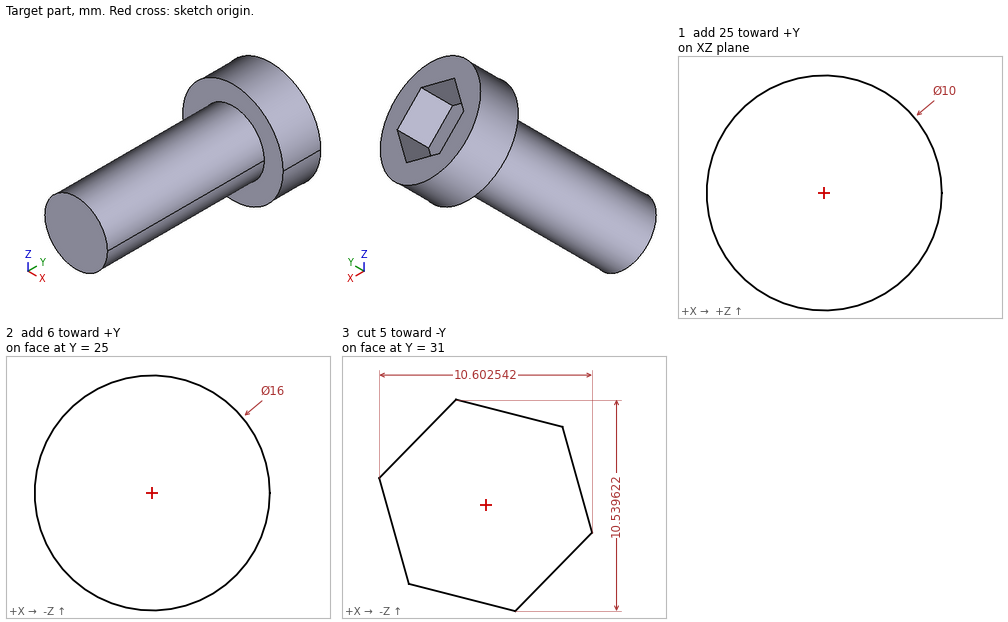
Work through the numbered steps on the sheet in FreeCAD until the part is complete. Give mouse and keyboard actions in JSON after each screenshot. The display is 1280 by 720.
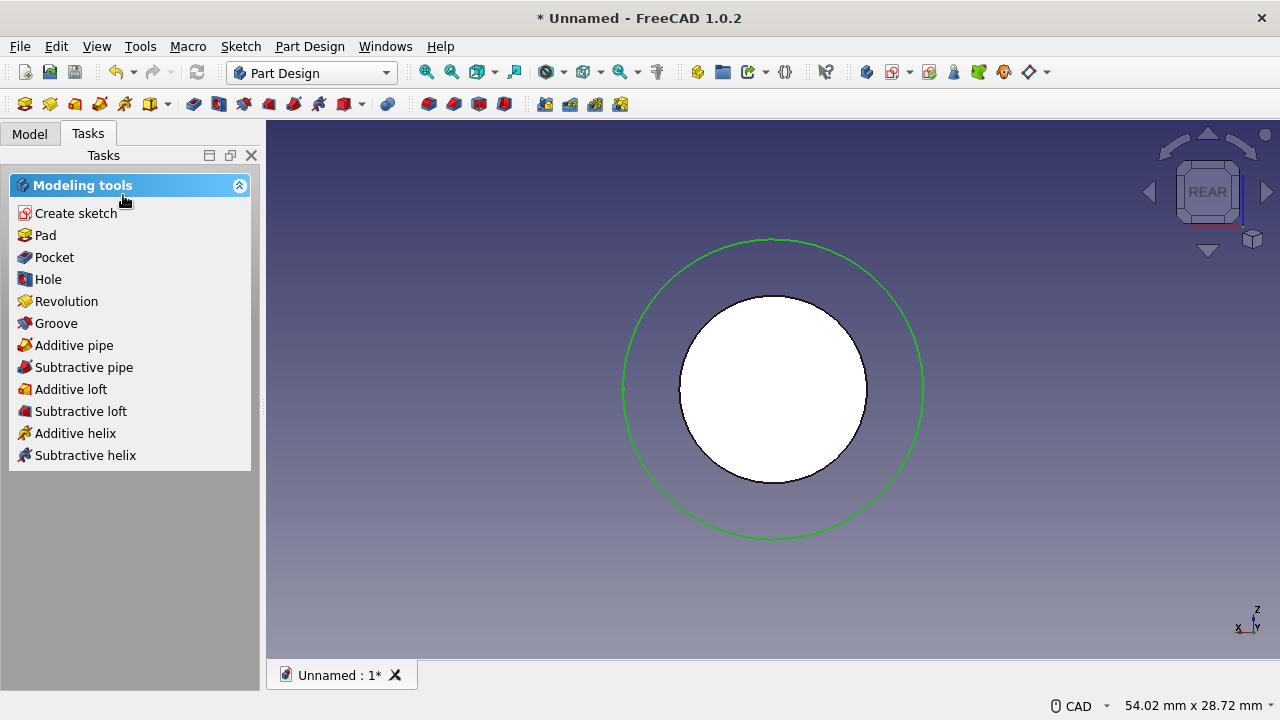
{"action": "left_click", "coordinate": [25, 104]}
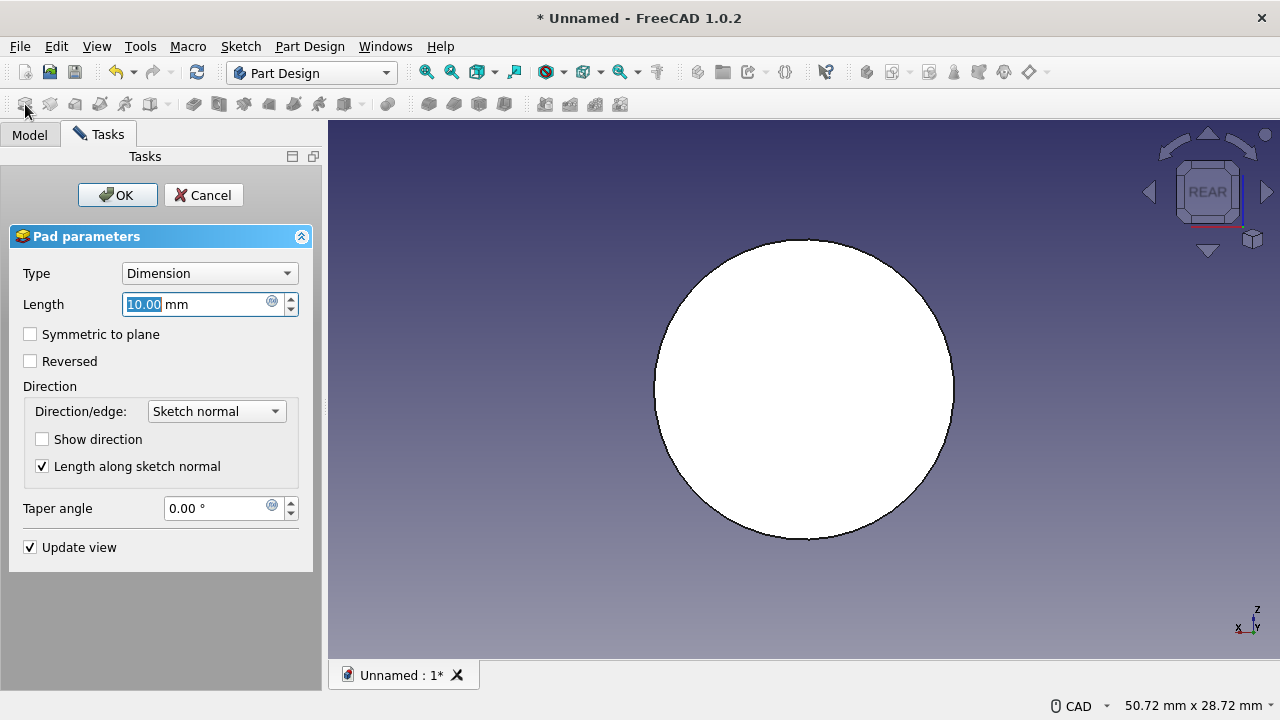
{"action": "type", "text": "6"}
{"action": "key", "text": "Tab"}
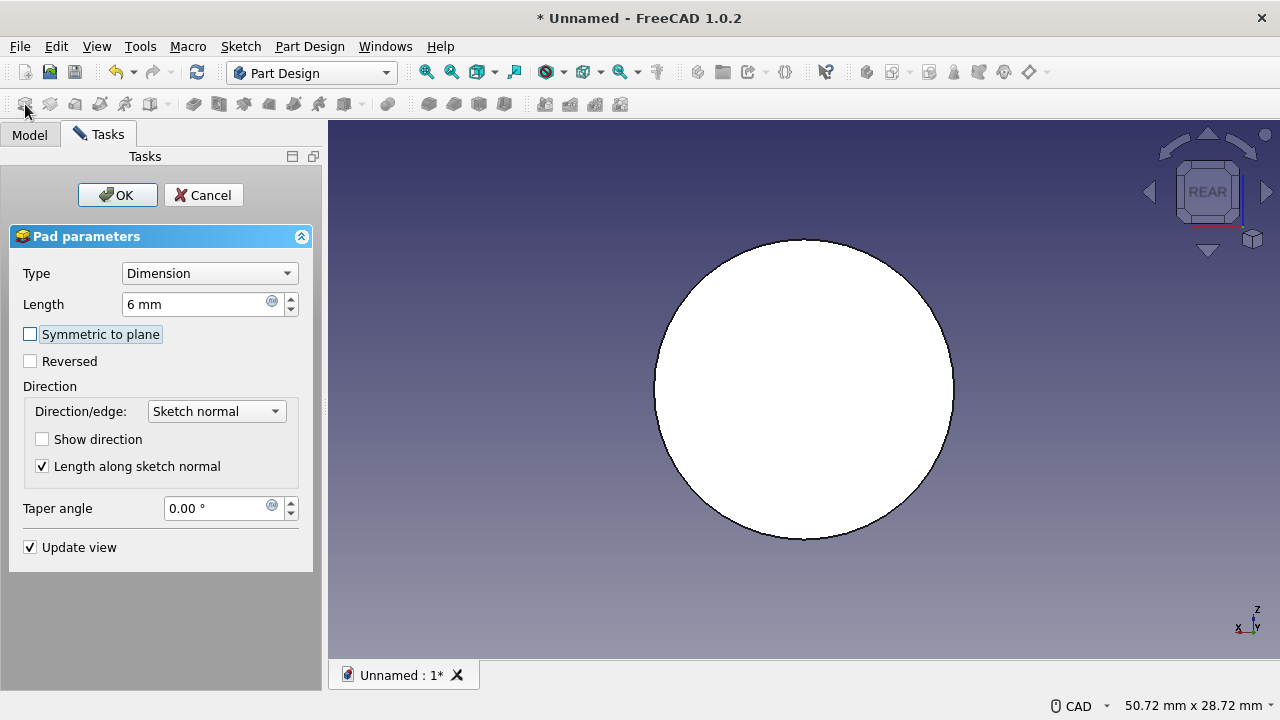
{"action": "left_click", "coordinate": [118, 195]}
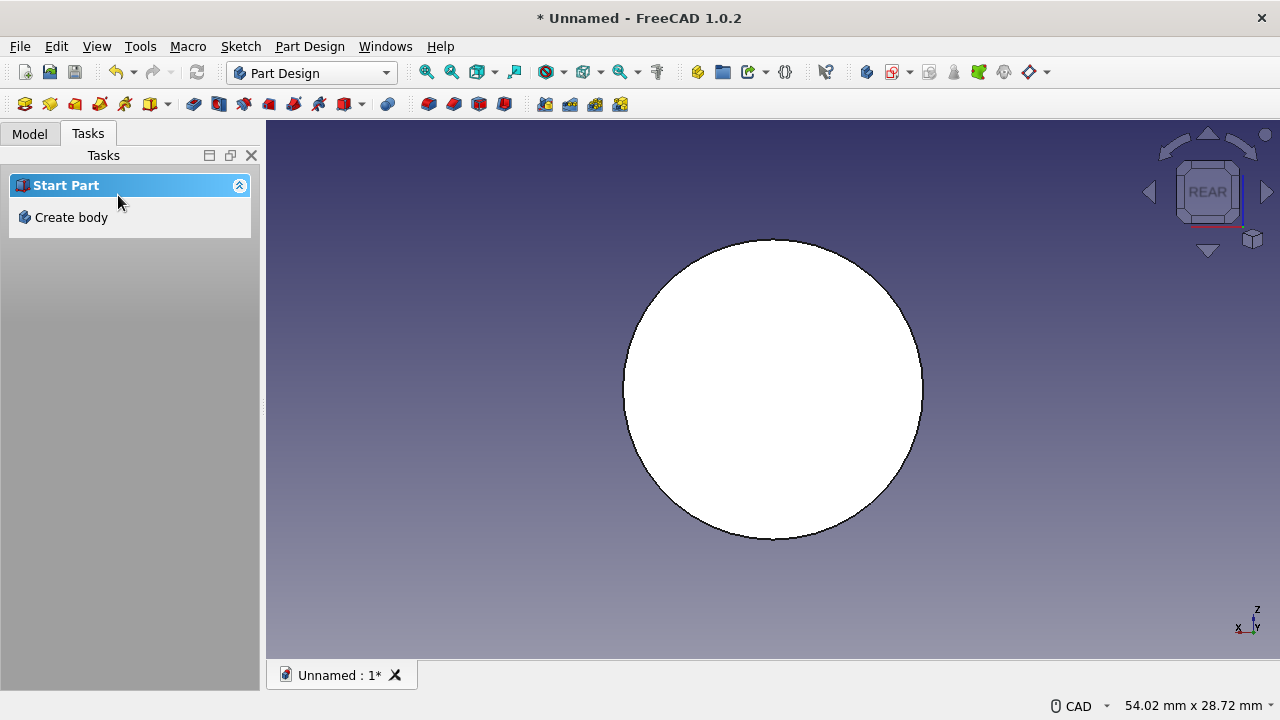
{"action": "left_click", "coordinate": [773, 389]}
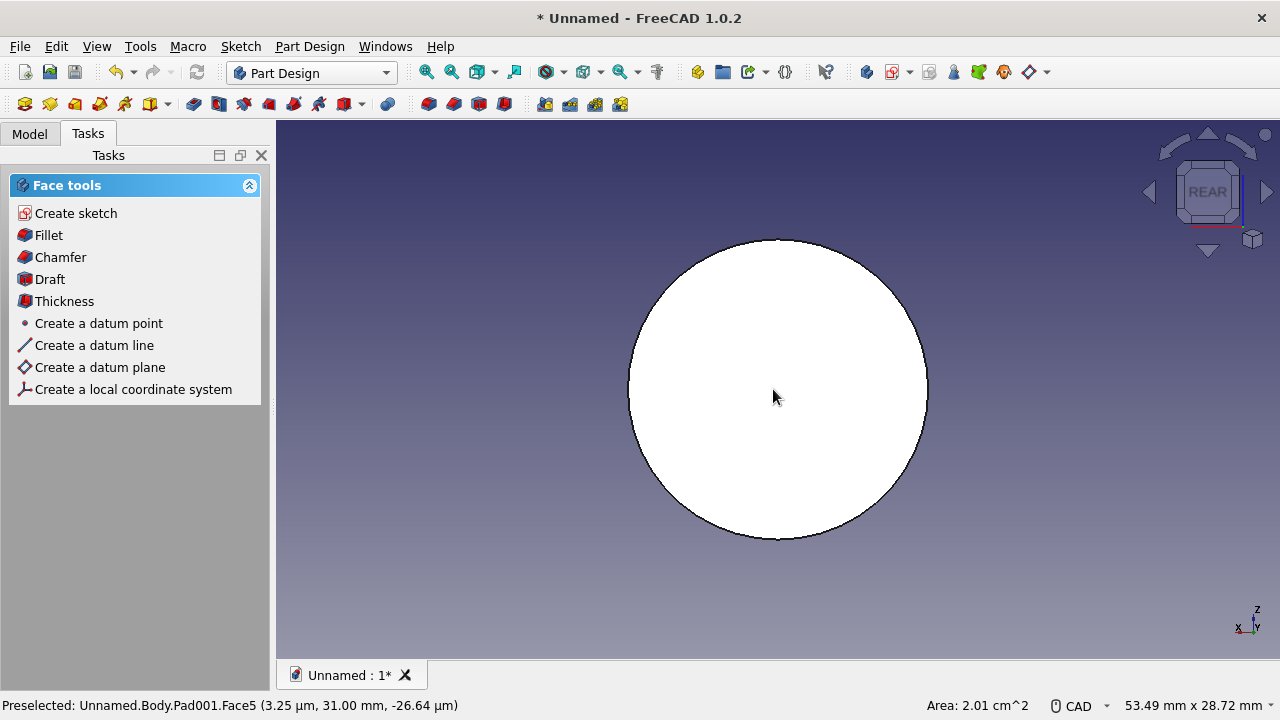
{"action": "left_click", "coordinate": [892, 72]}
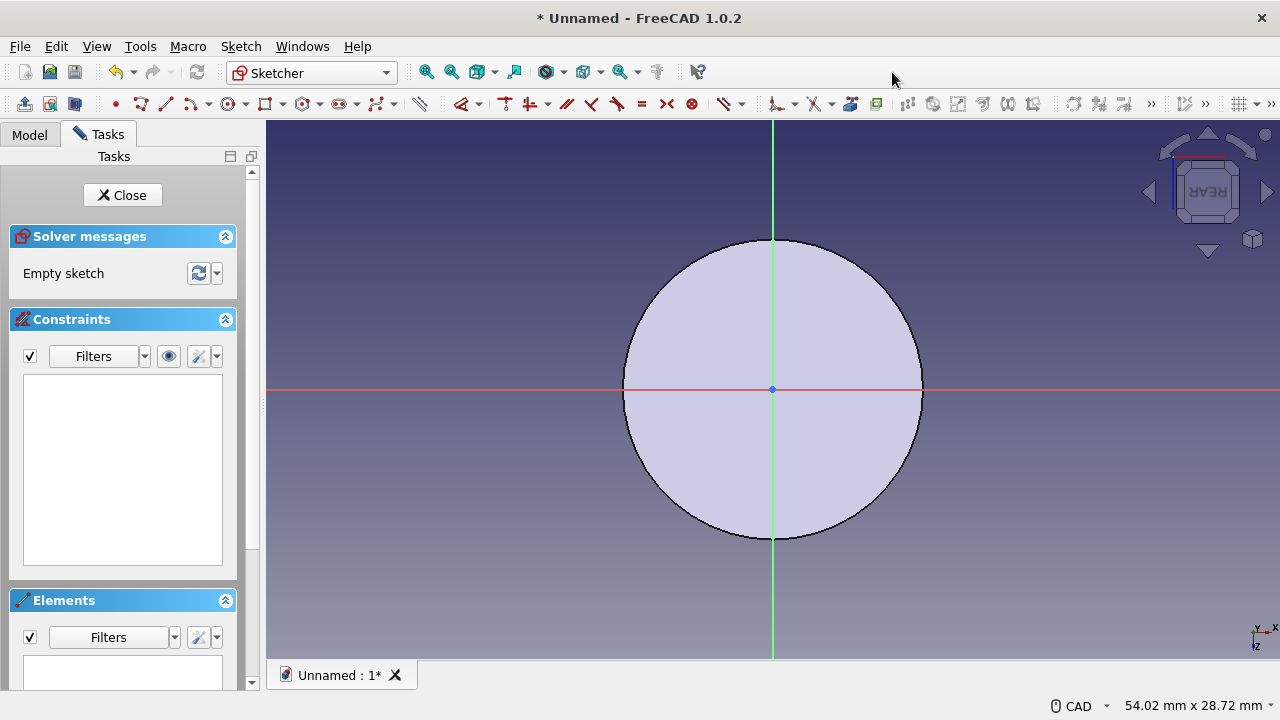
{"action": "scroll", "coordinate": [856, 389], "scroll_direction": "up", "scroll_amount": 3}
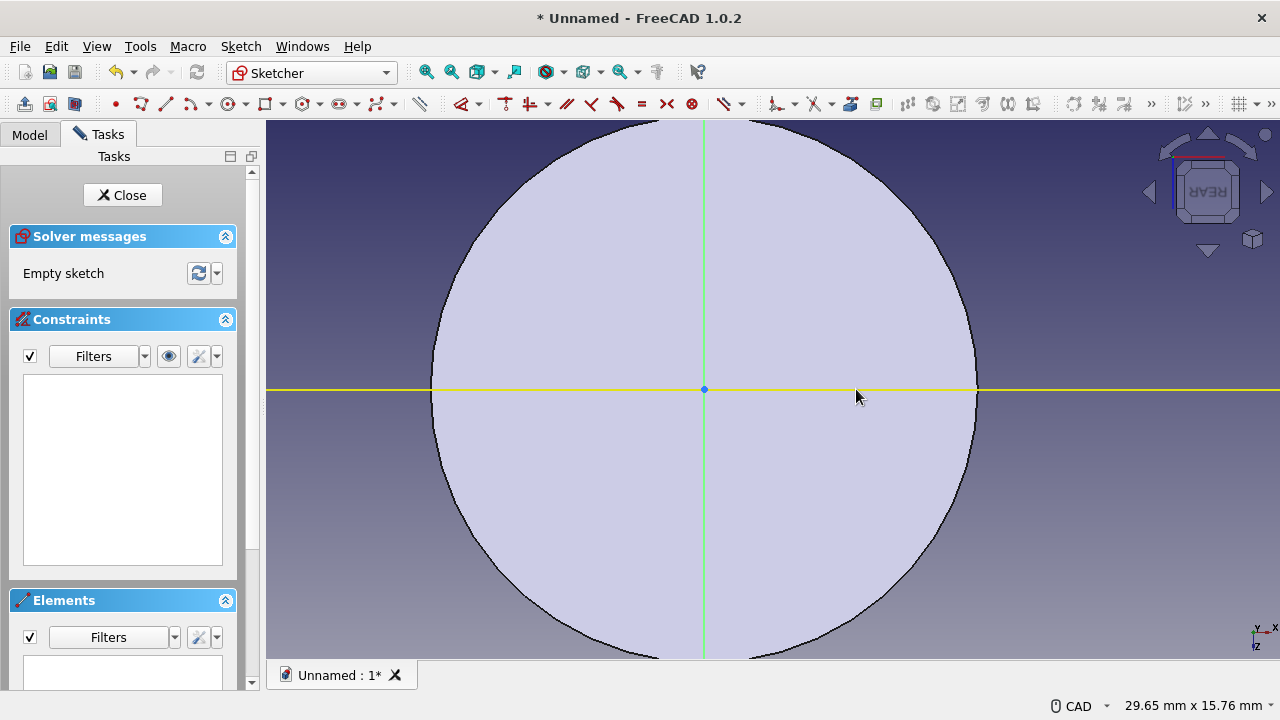
{"action": "key", "text": "g p 6"}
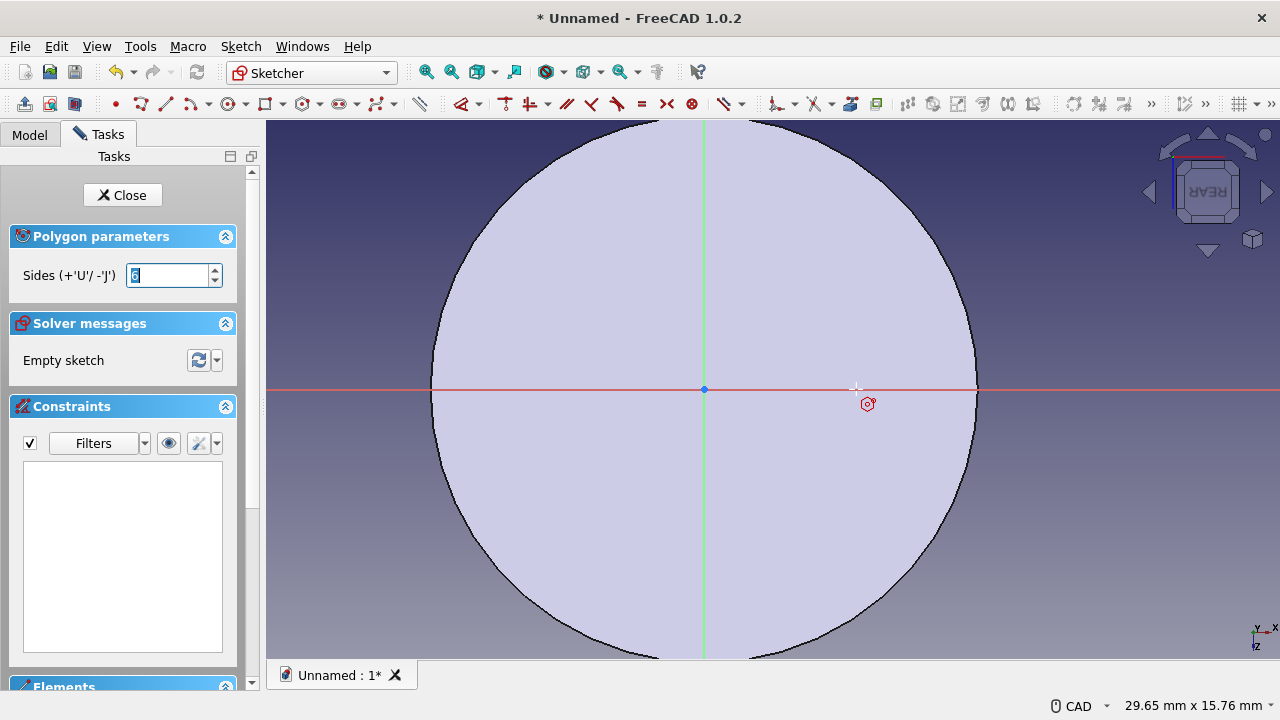
{"action": "left_click", "coordinate": [704, 389]}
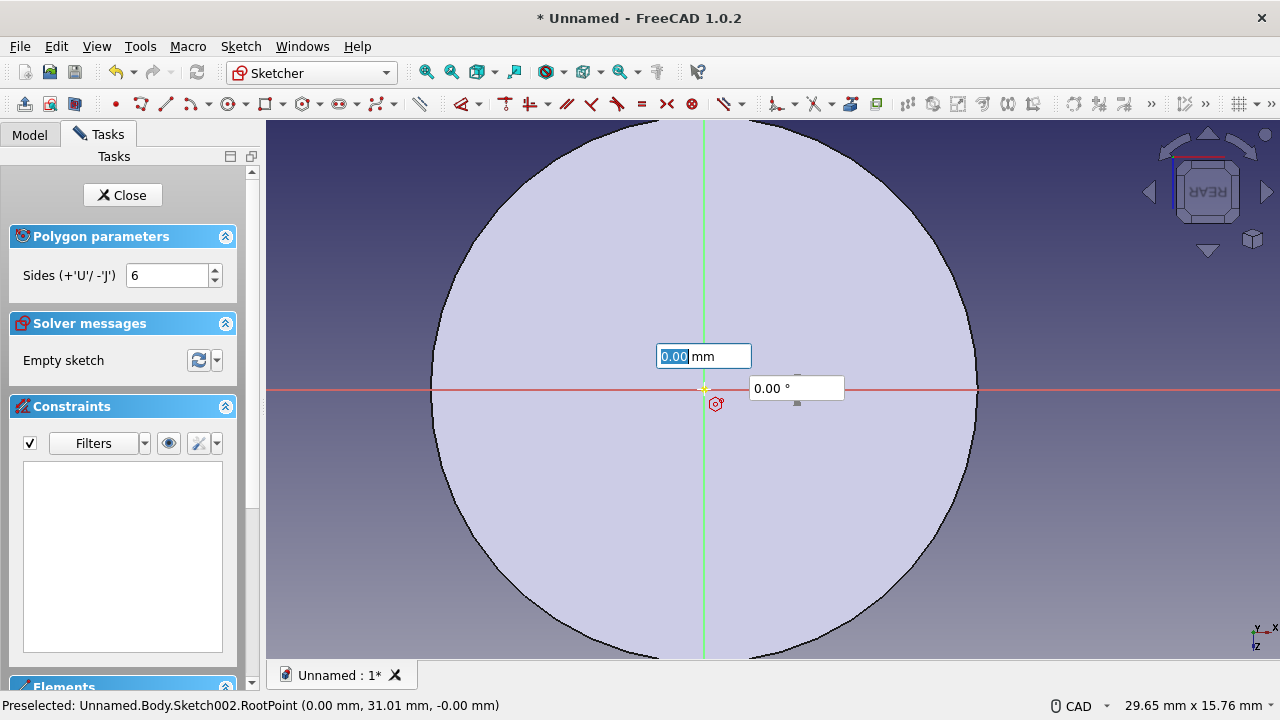
{"action": "left_click", "coordinate": [573, 523]}
{"action": "right_click", "coordinate": [573, 523]}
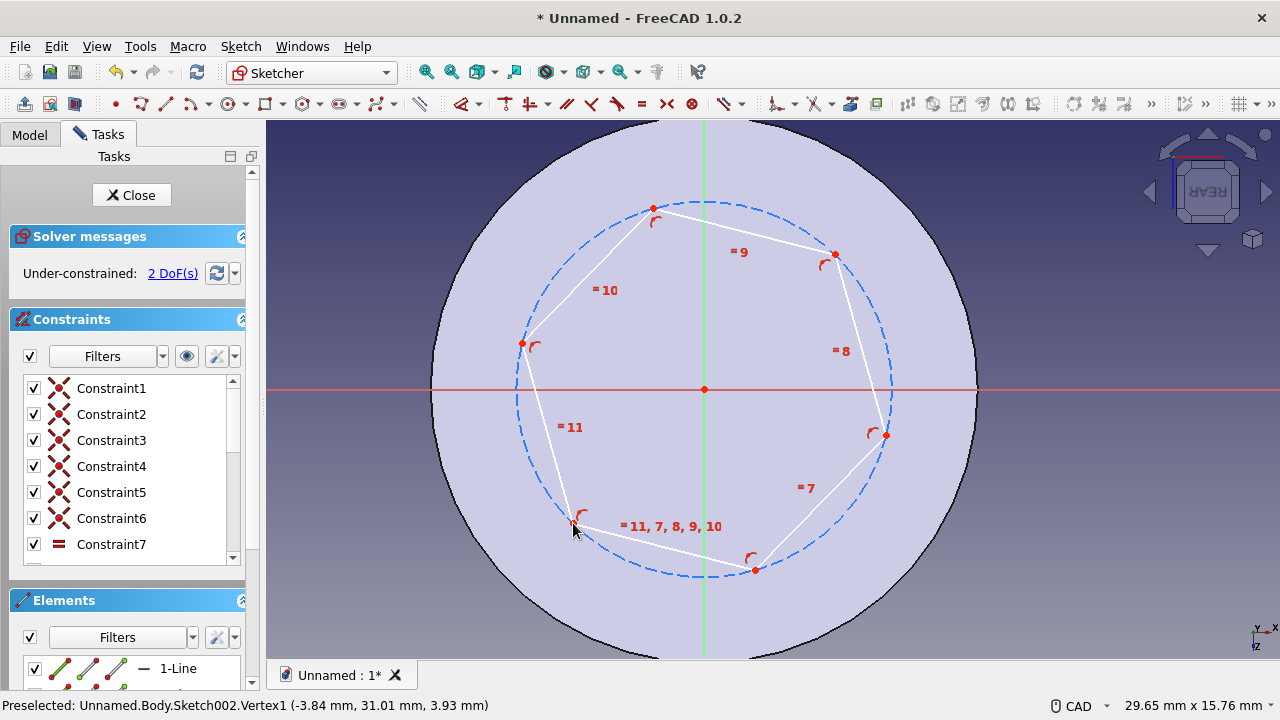
{"action": "key", "text": "d"}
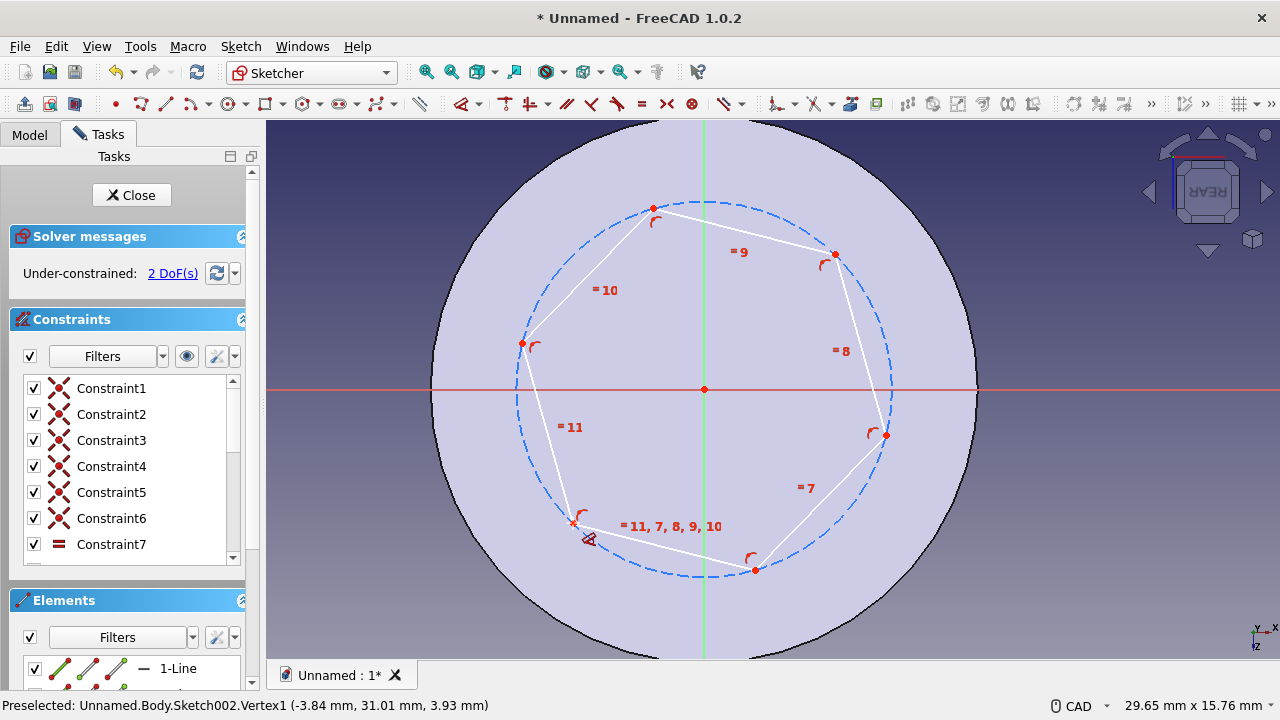
{"action": "left_click", "coordinate": [522, 343]}